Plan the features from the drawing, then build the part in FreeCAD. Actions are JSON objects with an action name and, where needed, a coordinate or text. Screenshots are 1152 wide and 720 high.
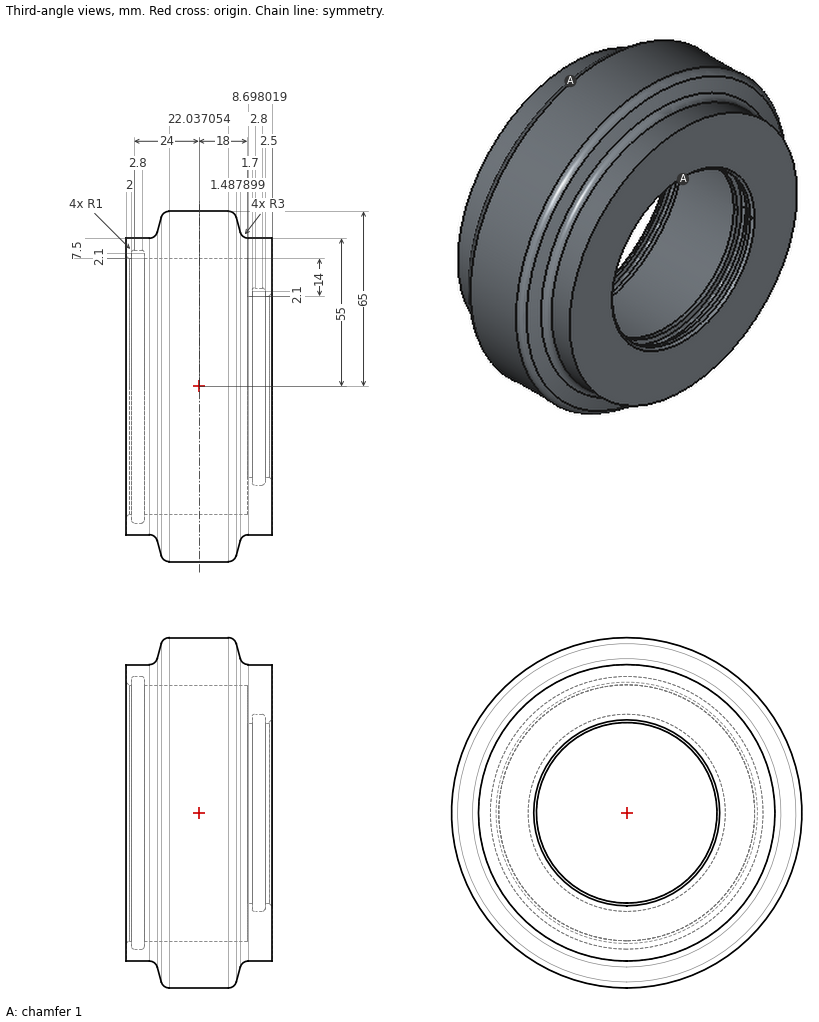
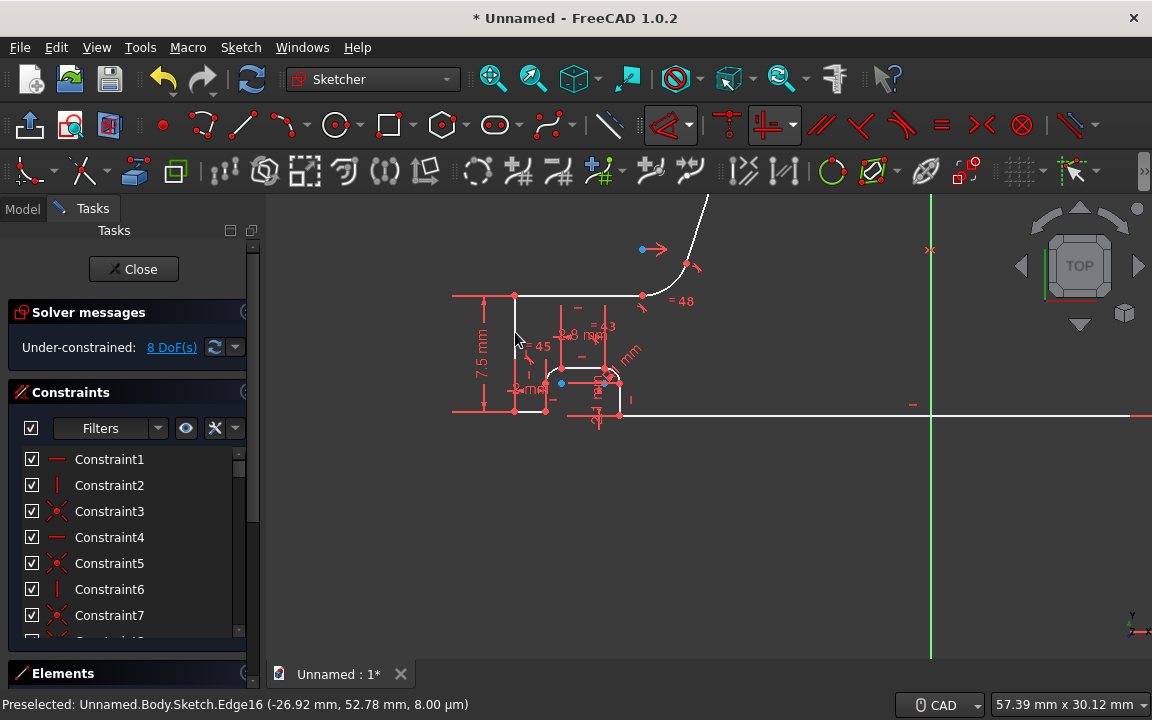
{"action": "scroll", "coordinate": [546, 400], "scroll_direction": "up", "scroll_amount": 2}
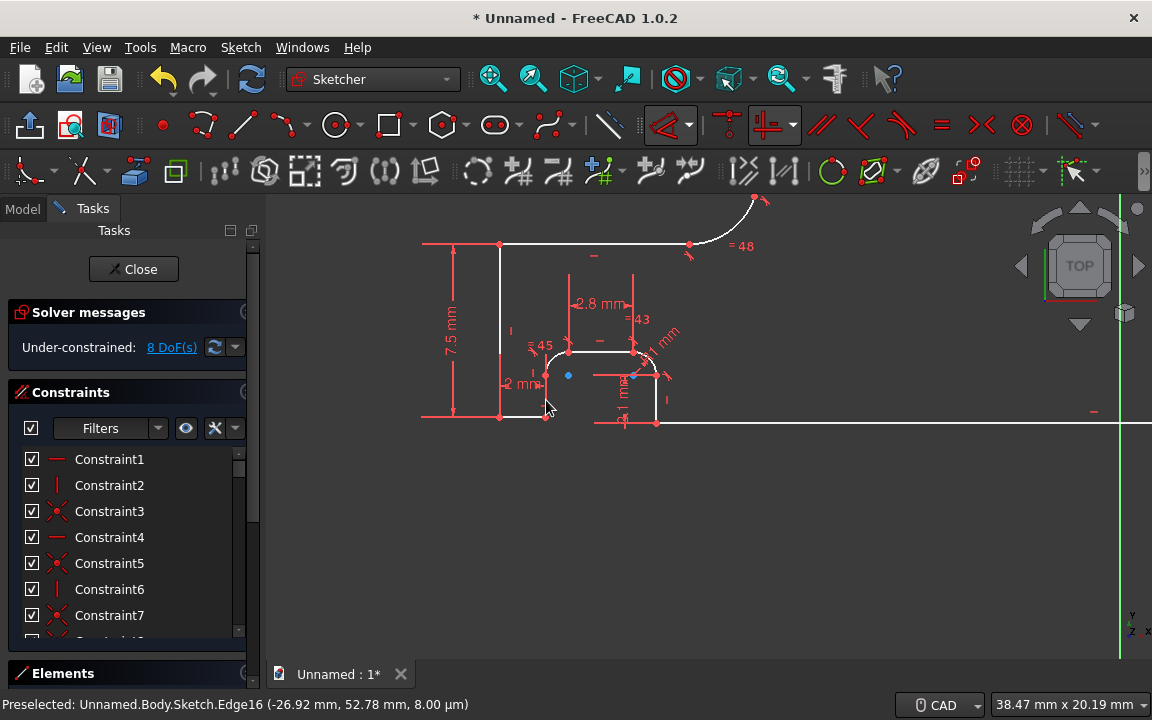
{"action": "left_click", "coordinate": [546, 392]}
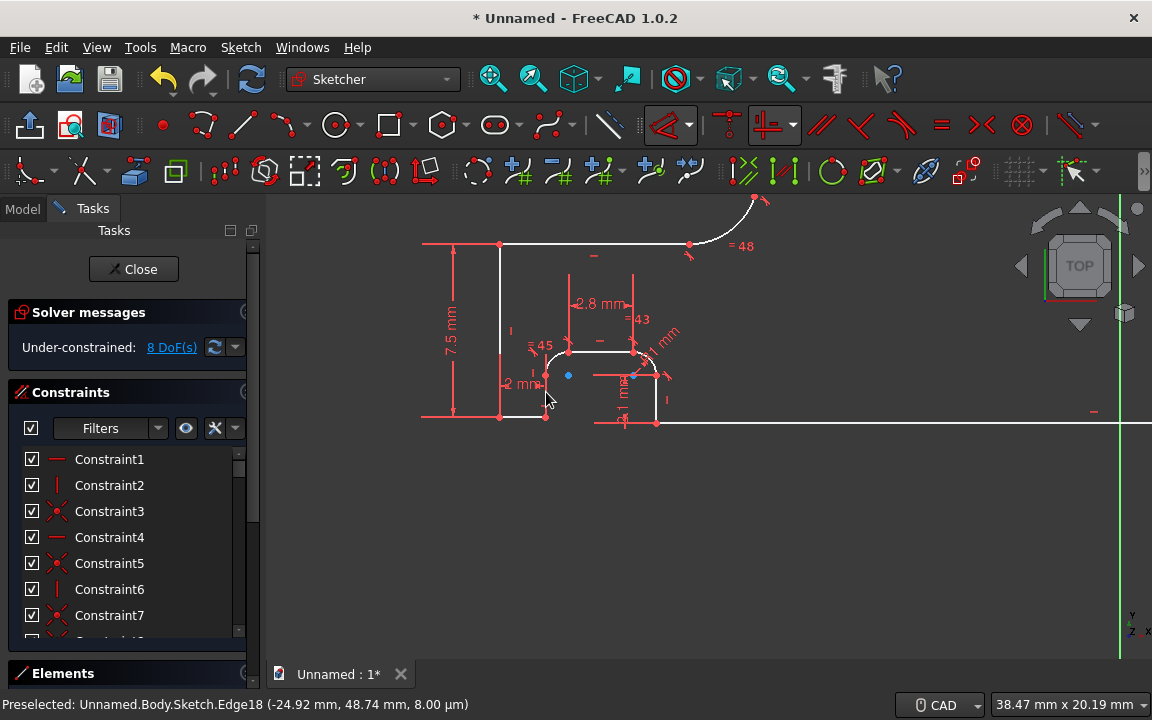
{"action": "key", "text": "i"}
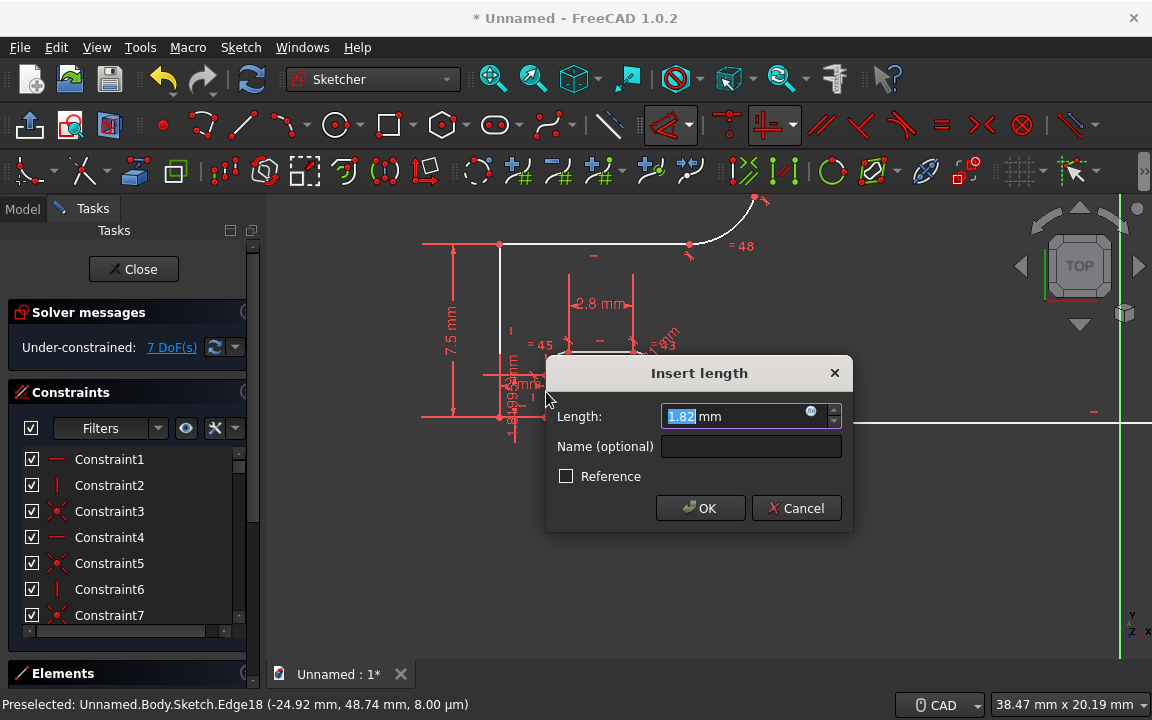
{"action": "type", "text": "2.1"}
{"action": "key", "text": "Return"}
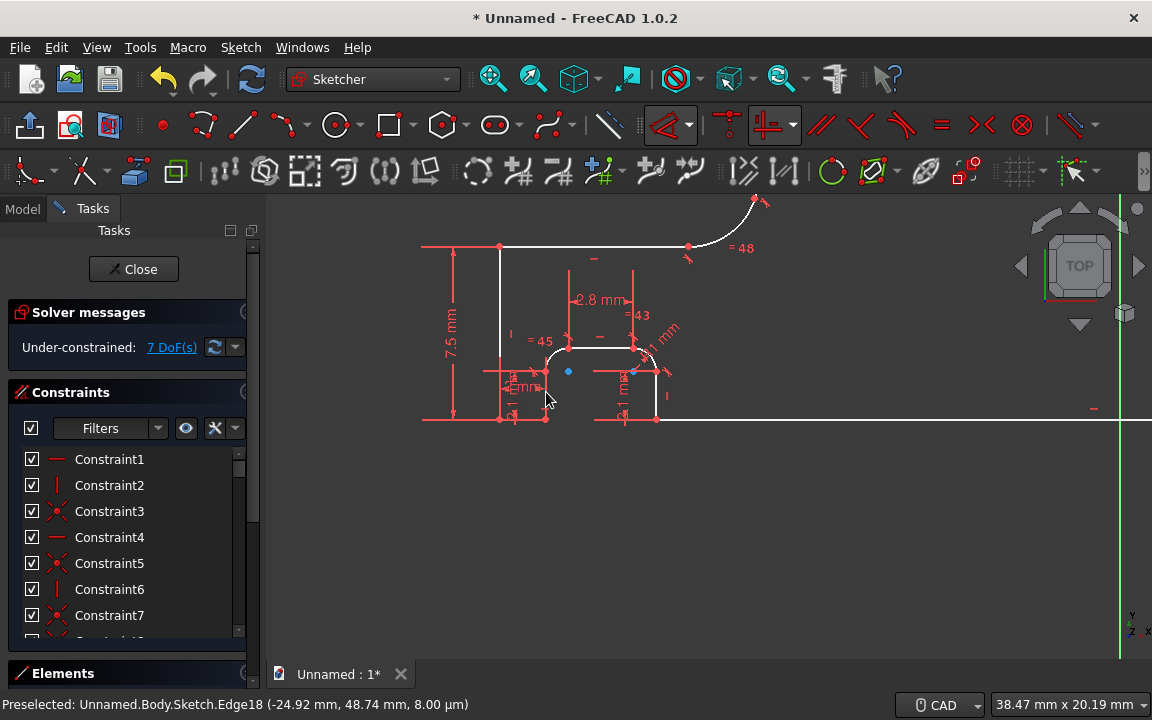
{"action": "left_click", "coordinate": [569, 348]}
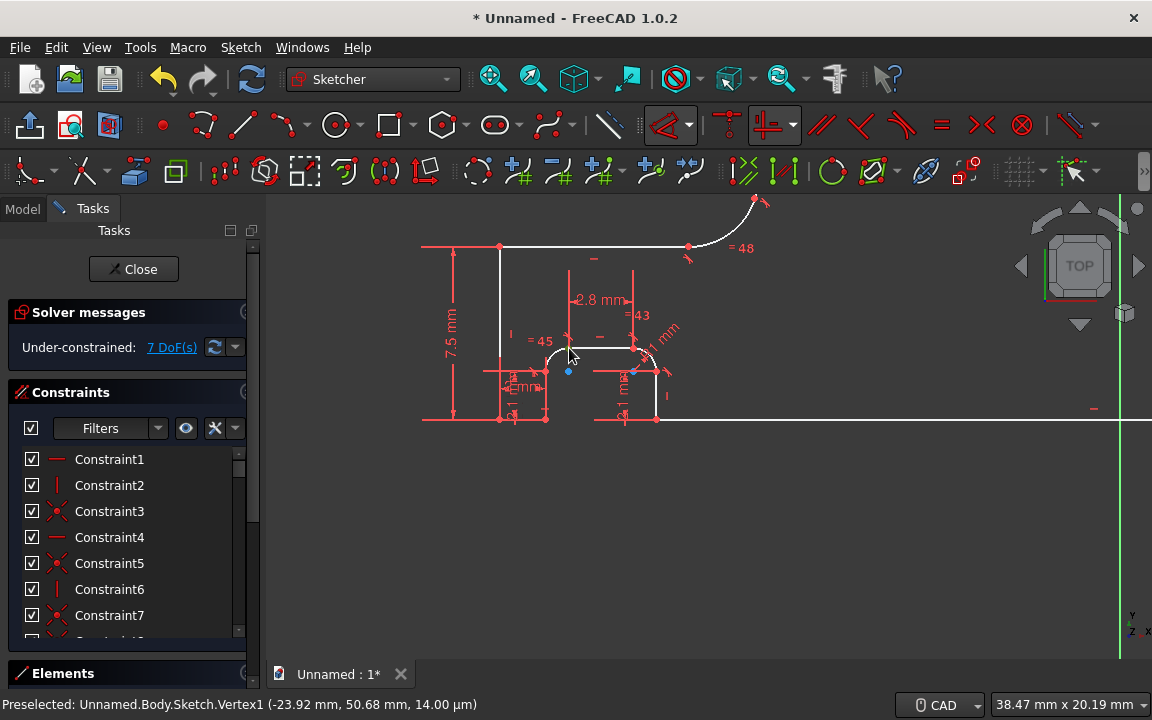
{"action": "key", "text": "l"}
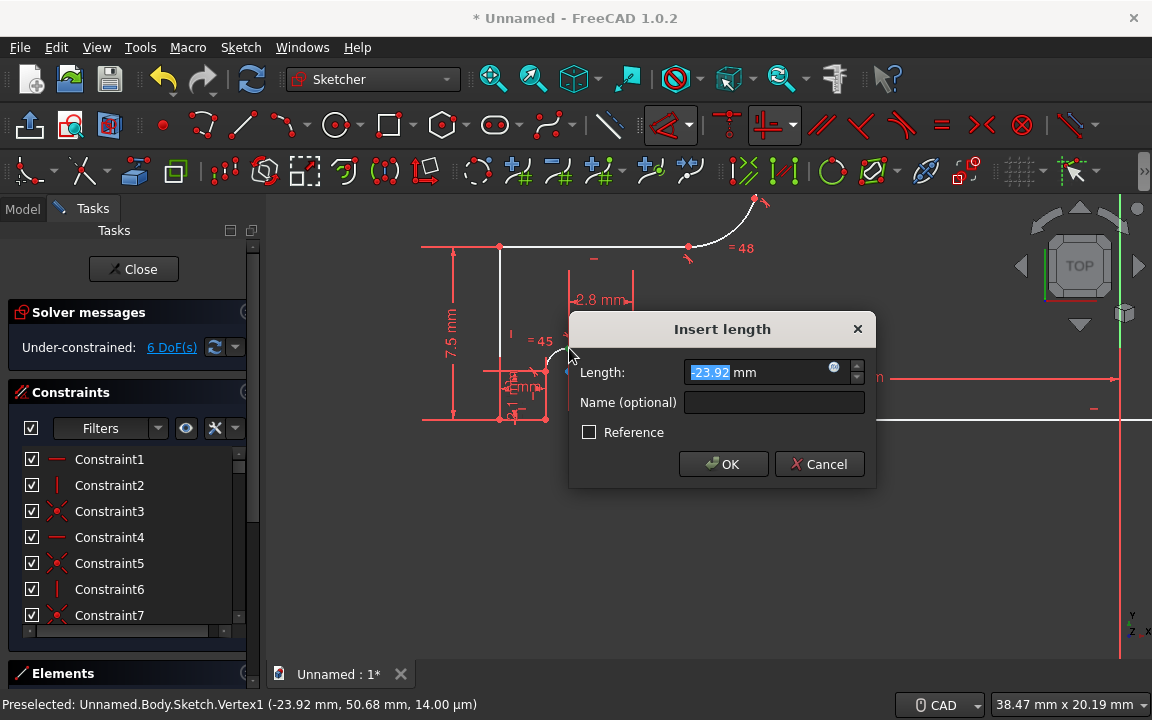
{"action": "type", "text": "-24"}
{"action": "key", "text": "Return"}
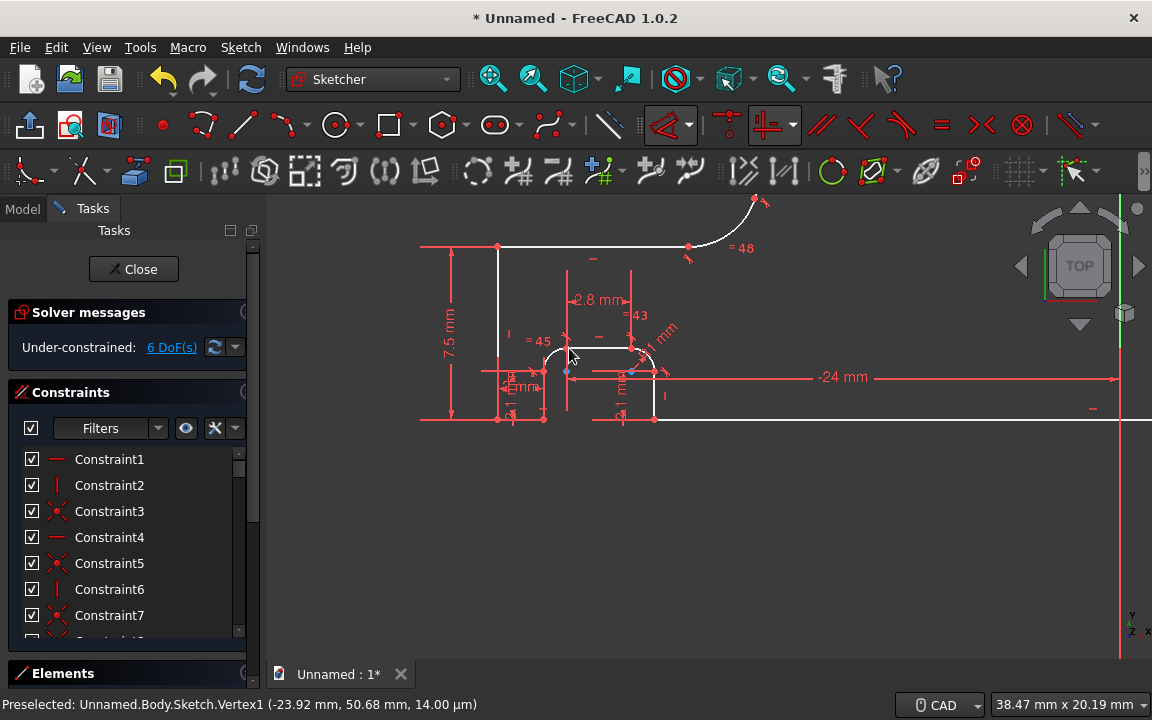
{"action": "scroll", "coordinate": [519, 340], "scroll_direction": "down", "scroll_amount": 8}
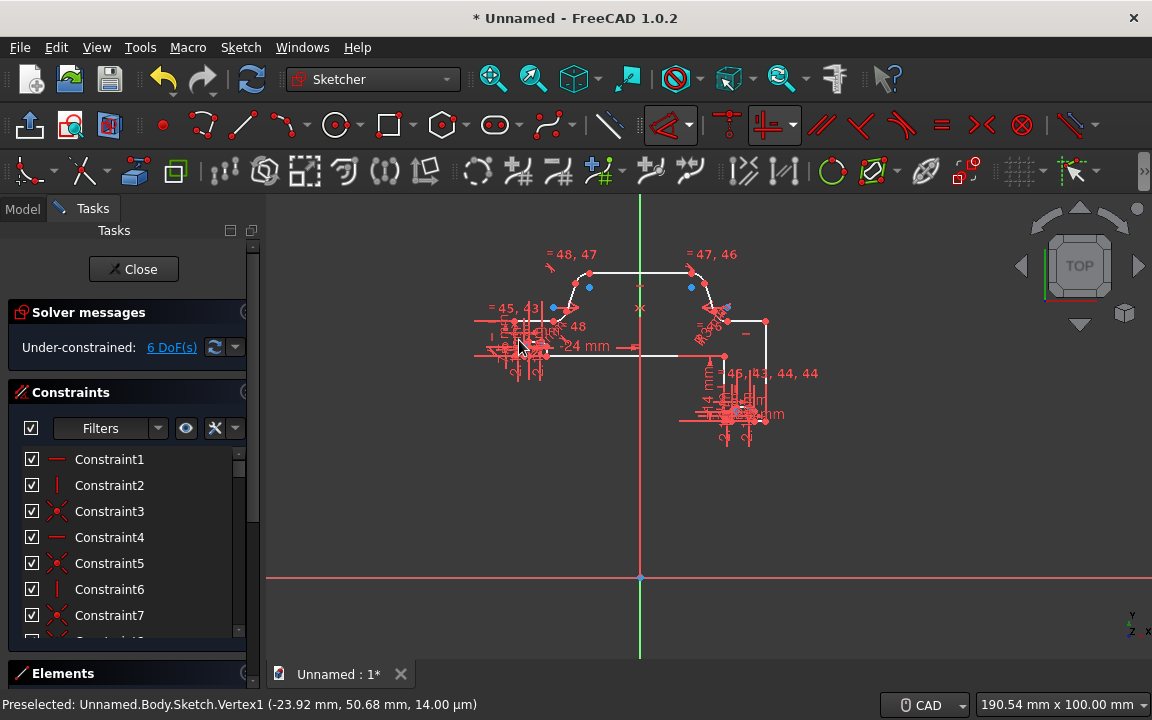
{"action": "left_click", "coordinate": [724, 356]}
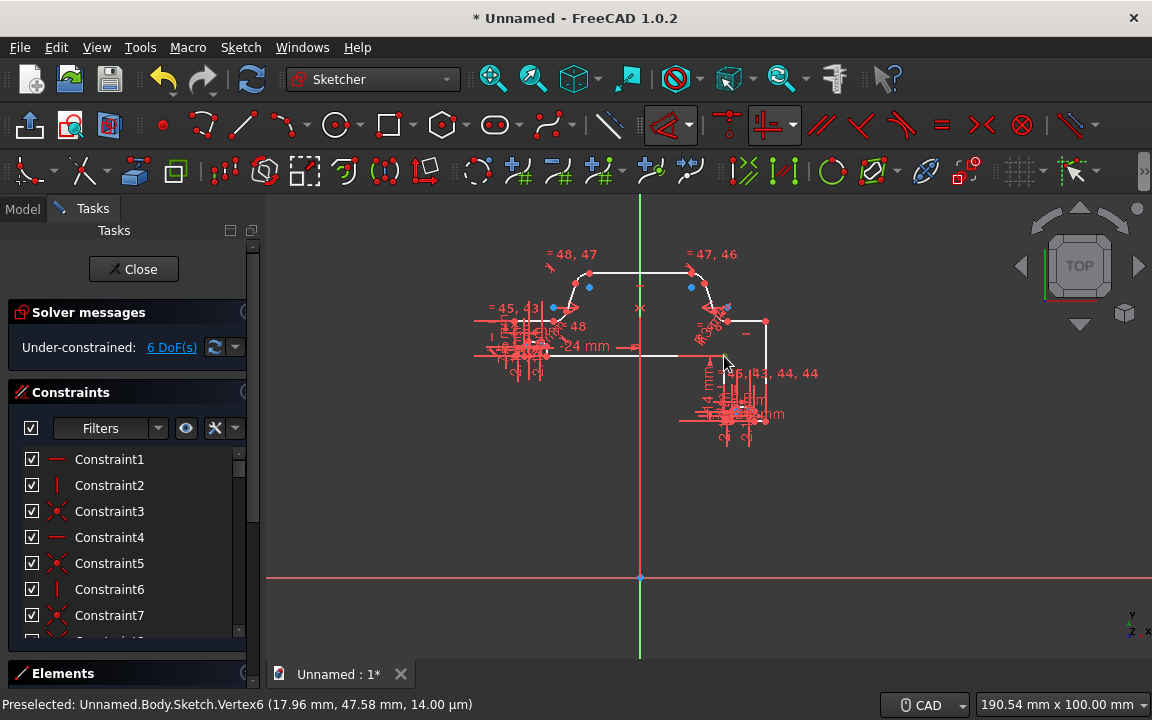
{"action": "key", "text": "l"}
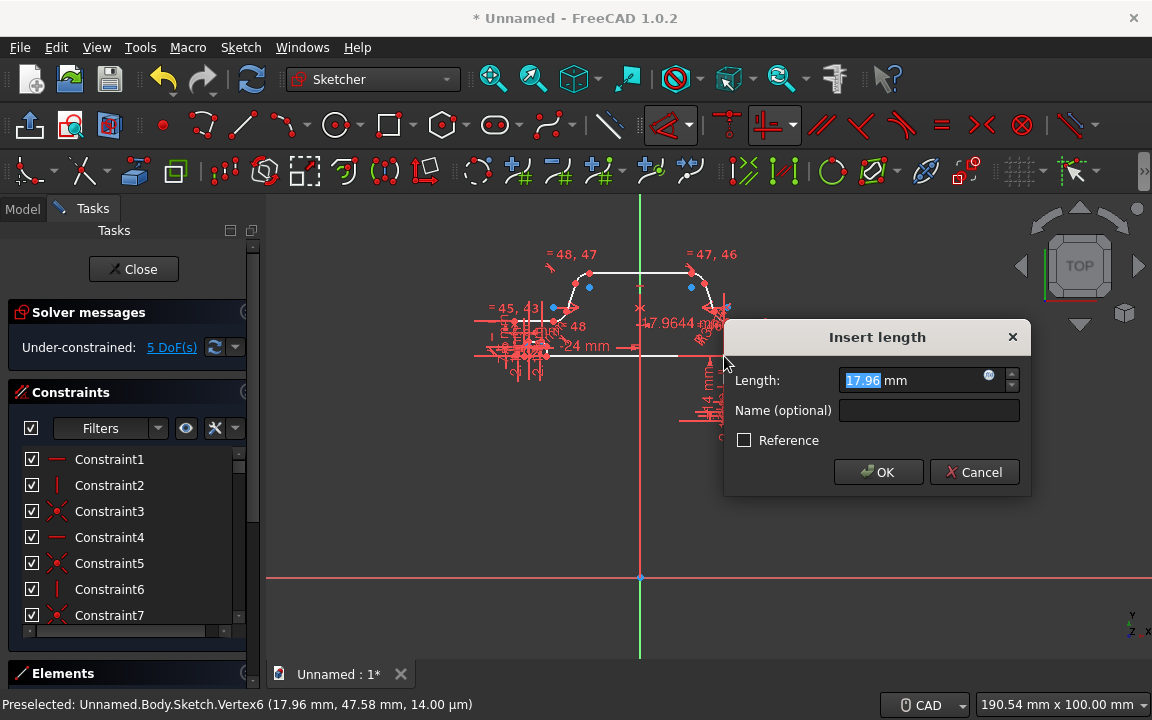
{"action": "type", "text": "18"}
{"action": "key", "text": "Return"}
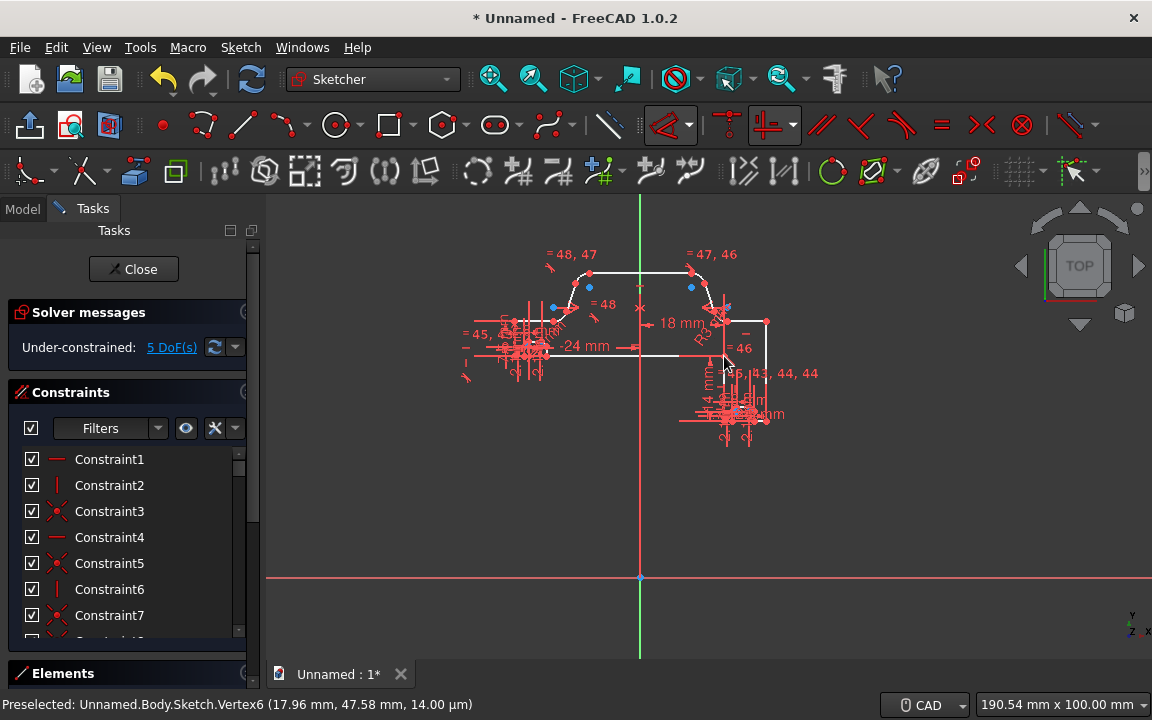
{"action": "left_click", "coordinate": [766, 321]}